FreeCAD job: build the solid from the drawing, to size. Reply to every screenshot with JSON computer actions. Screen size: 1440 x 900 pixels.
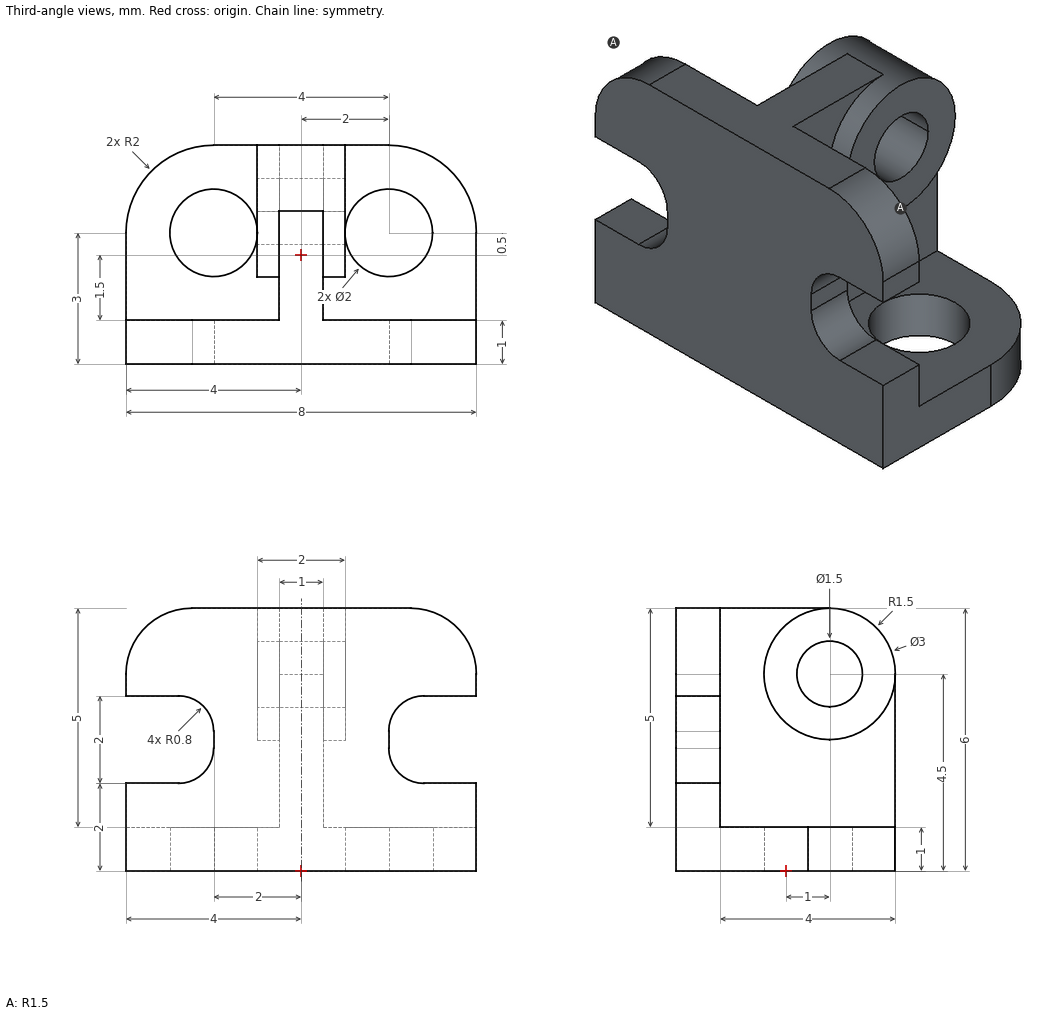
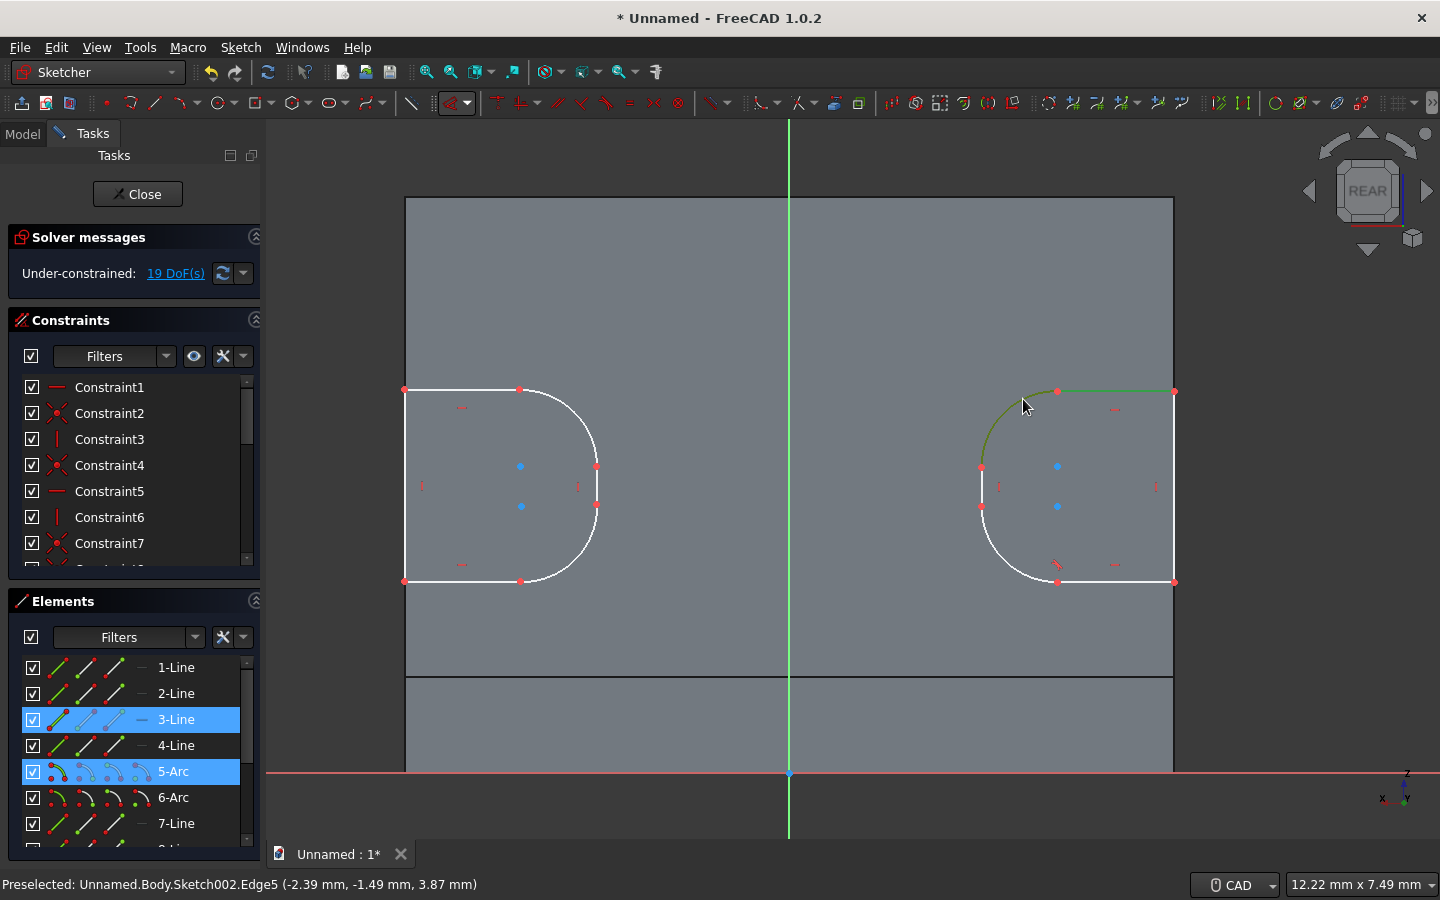
{"action": "left_click", "coordinate": [606, 104]}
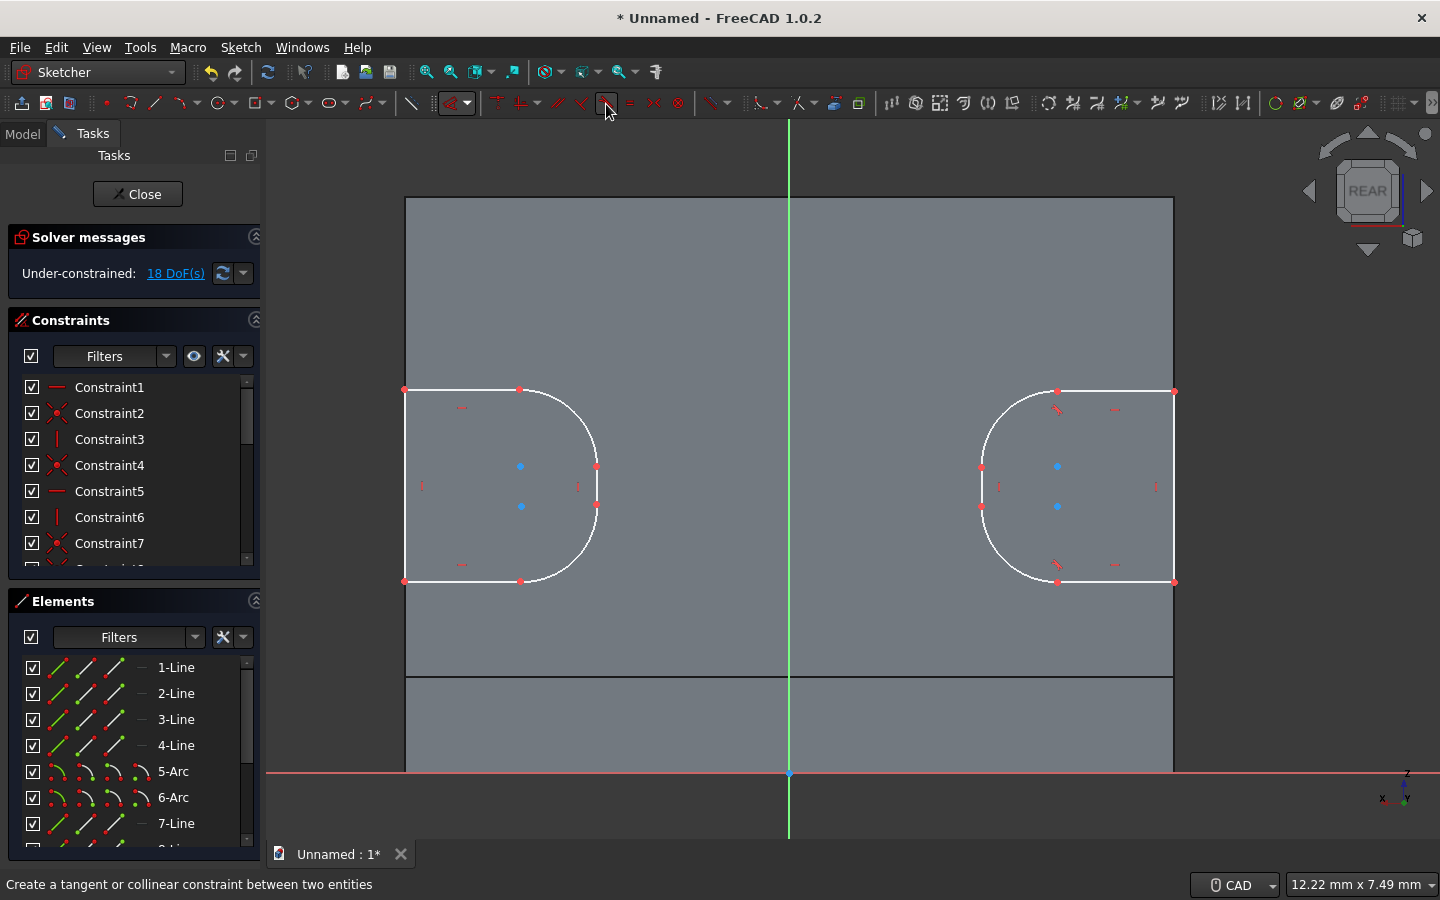
{"action": "left_click", "coordinate": [982, 479]}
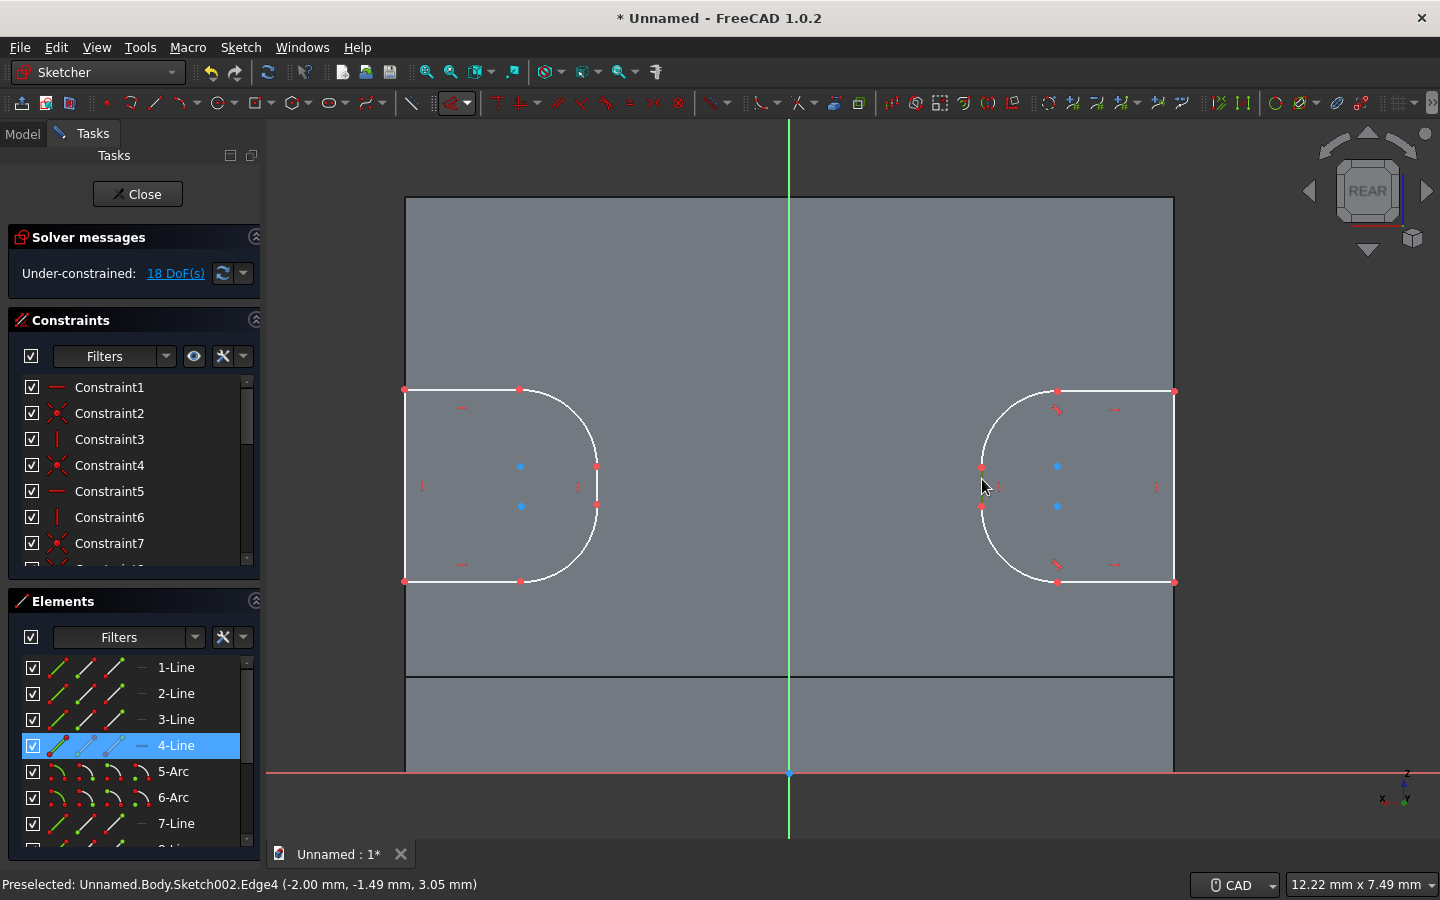
{"action": "left_click", "coordinate": [1023, 399]}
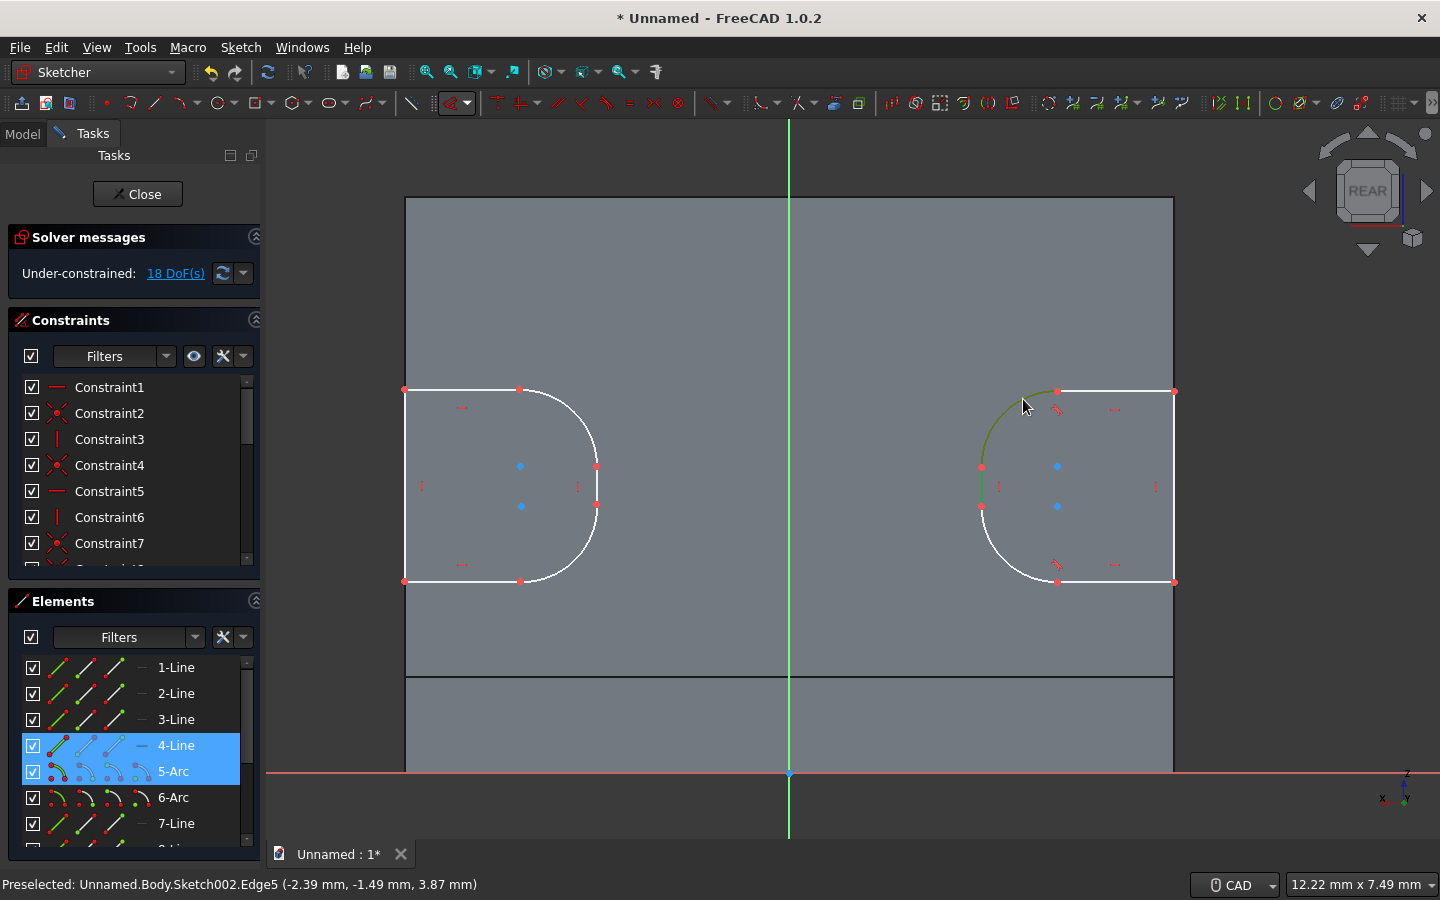
{"action": "key", "text": "t"}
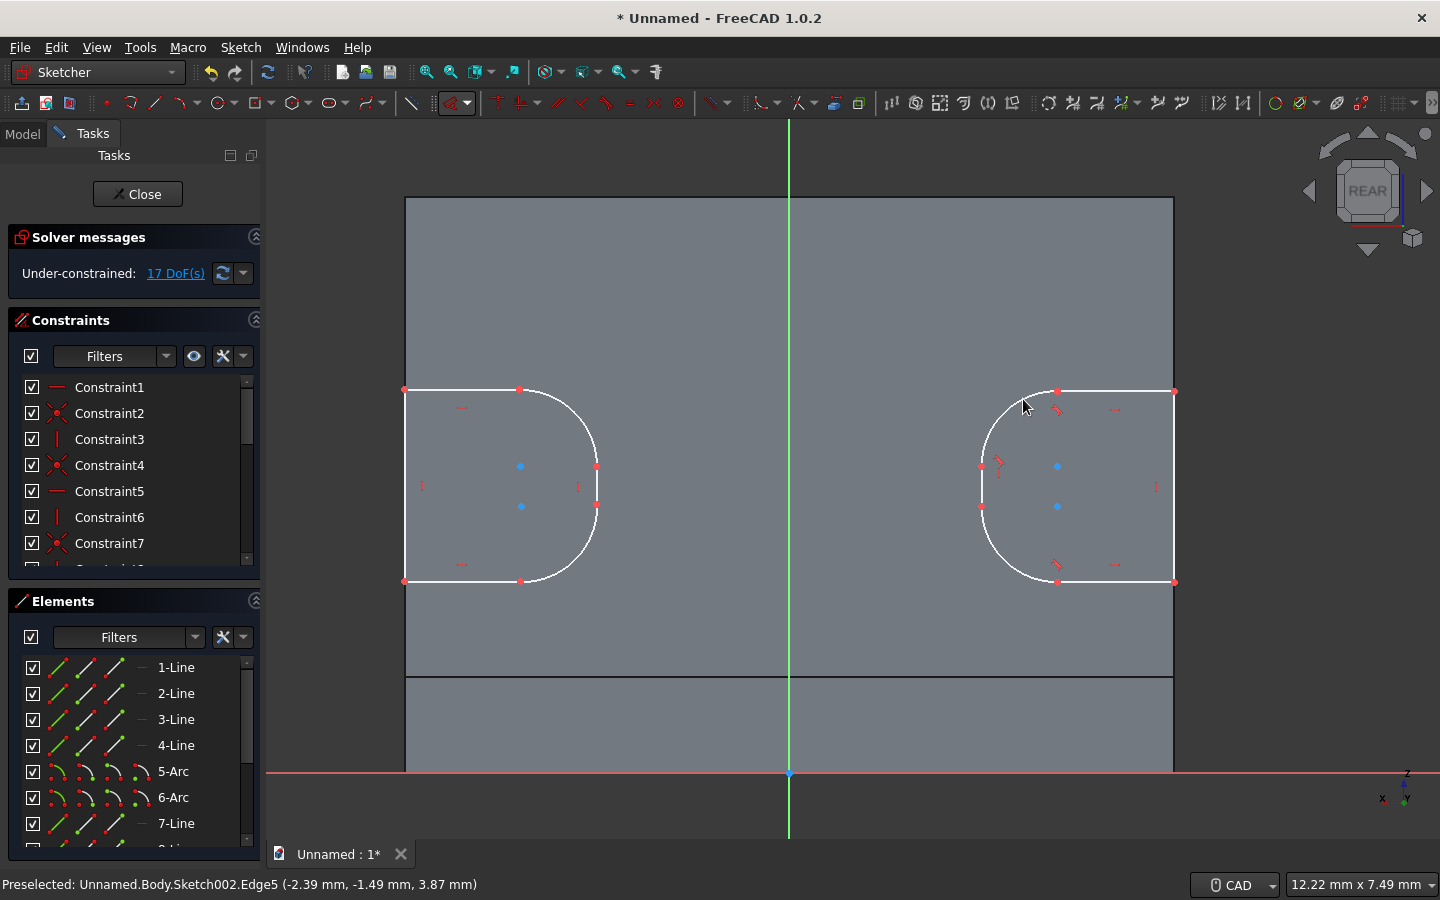
{"action": "left_click", "coordinate": [982, 478]}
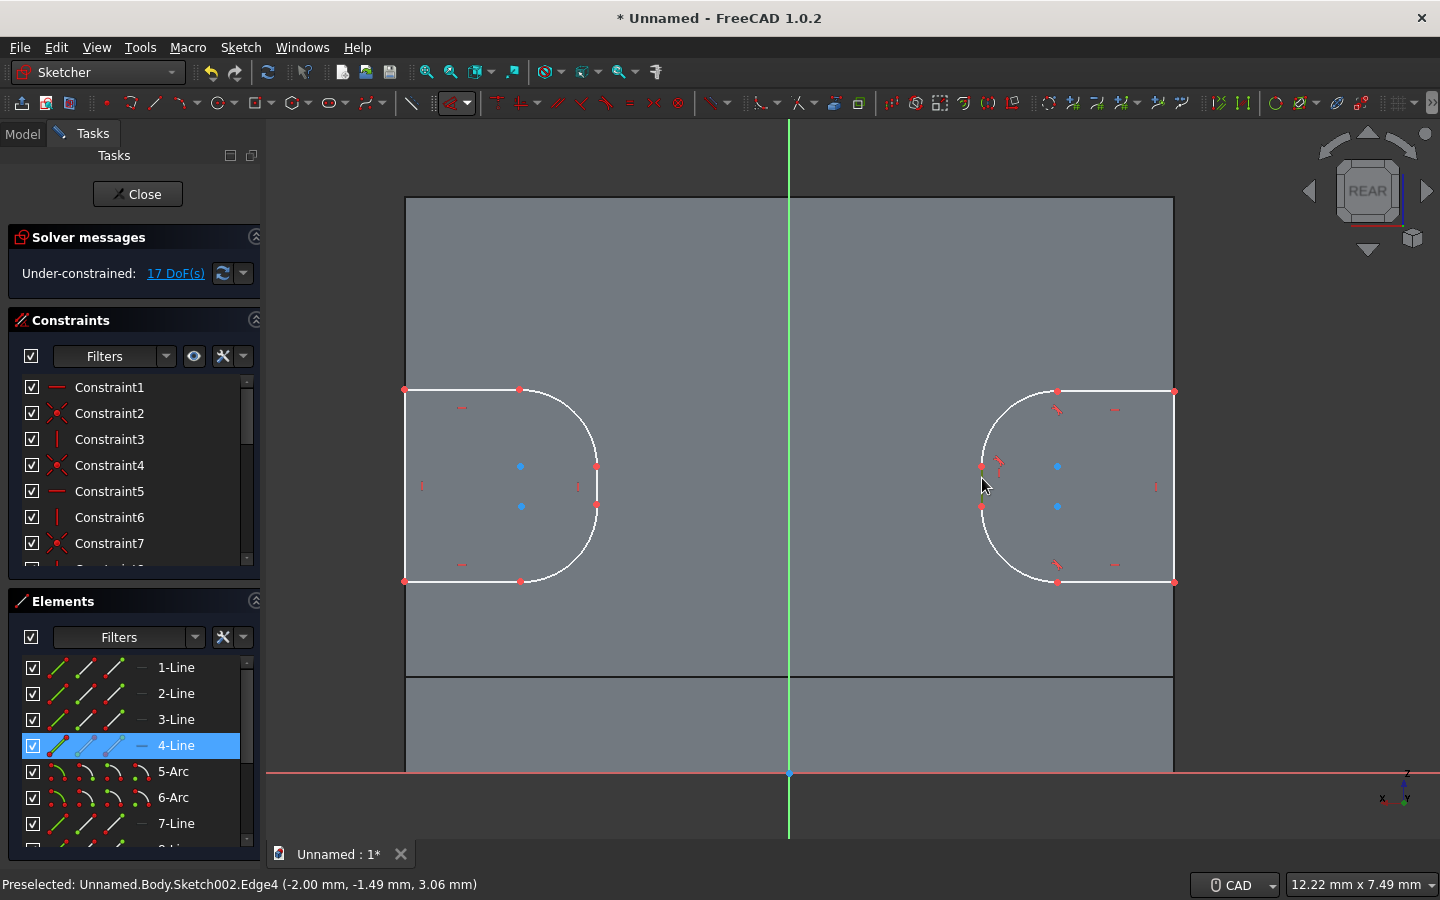
{"action": "left_click", "coordinate": [990, 541]}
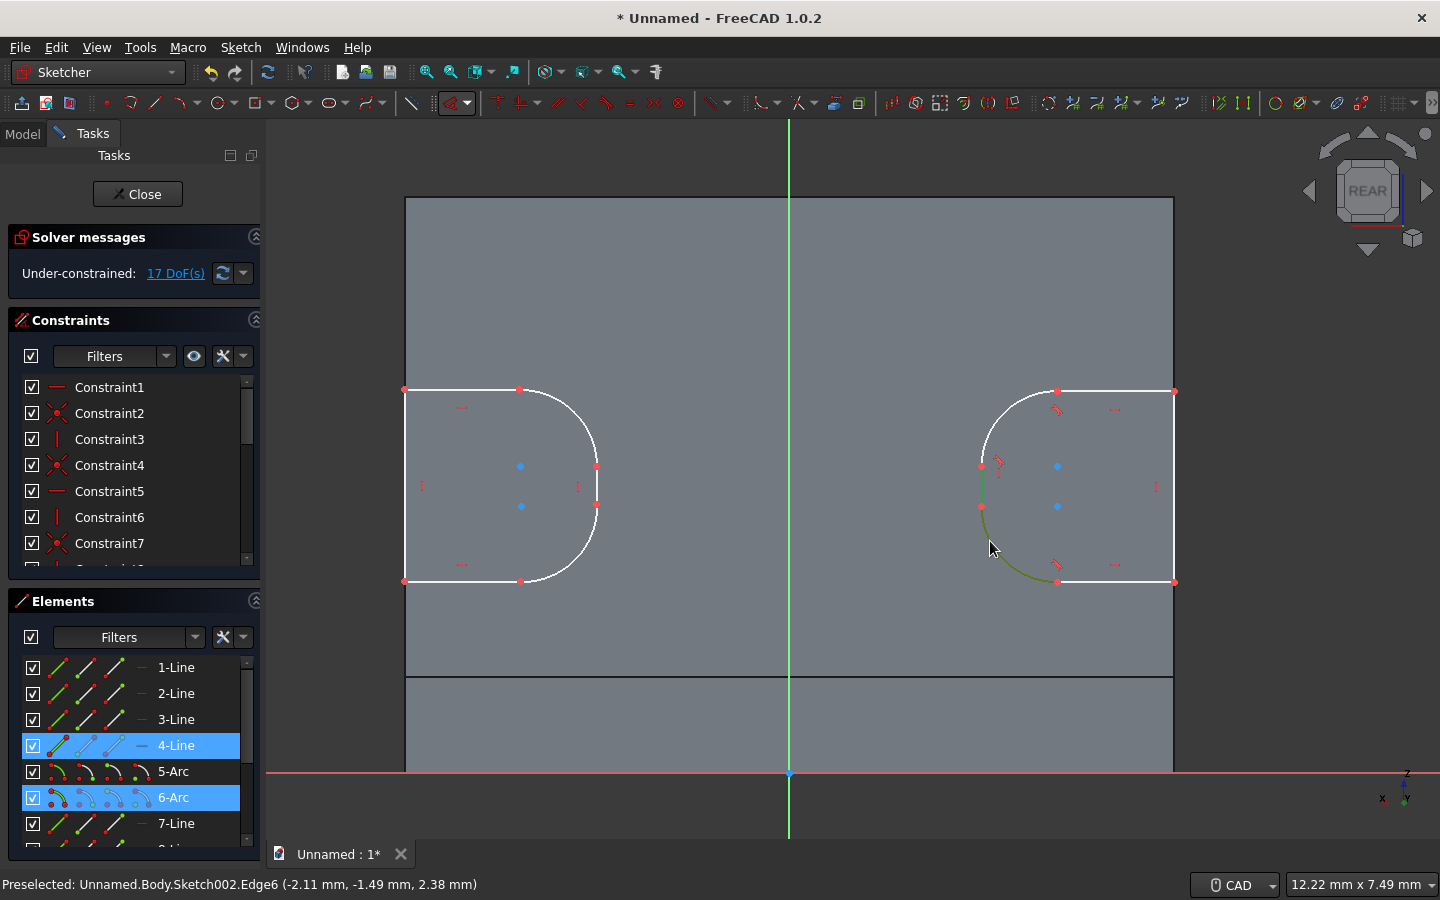
{"action": "left_click", "coordinate": [606, 104]}